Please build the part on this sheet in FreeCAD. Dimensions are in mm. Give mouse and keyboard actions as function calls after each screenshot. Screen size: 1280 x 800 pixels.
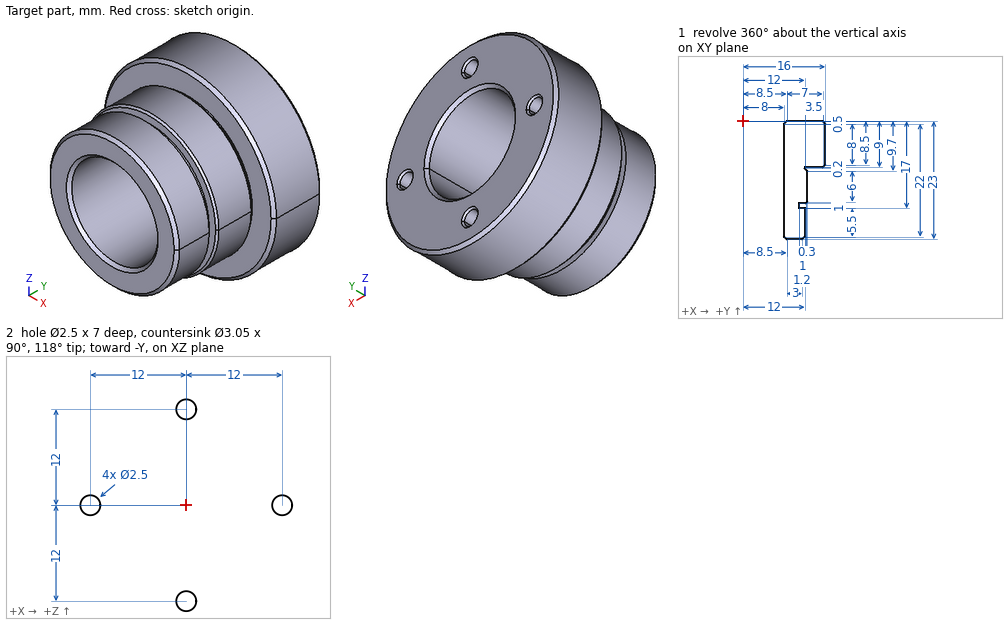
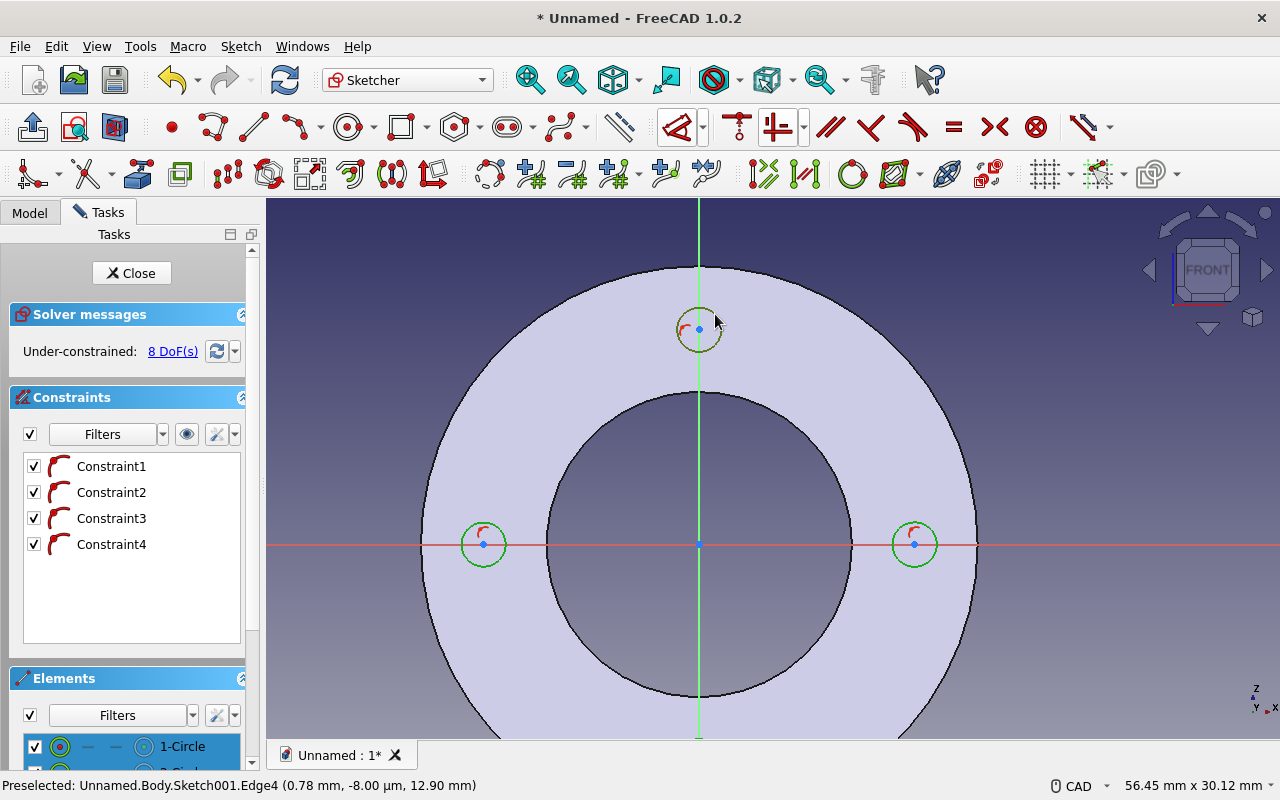
key(e)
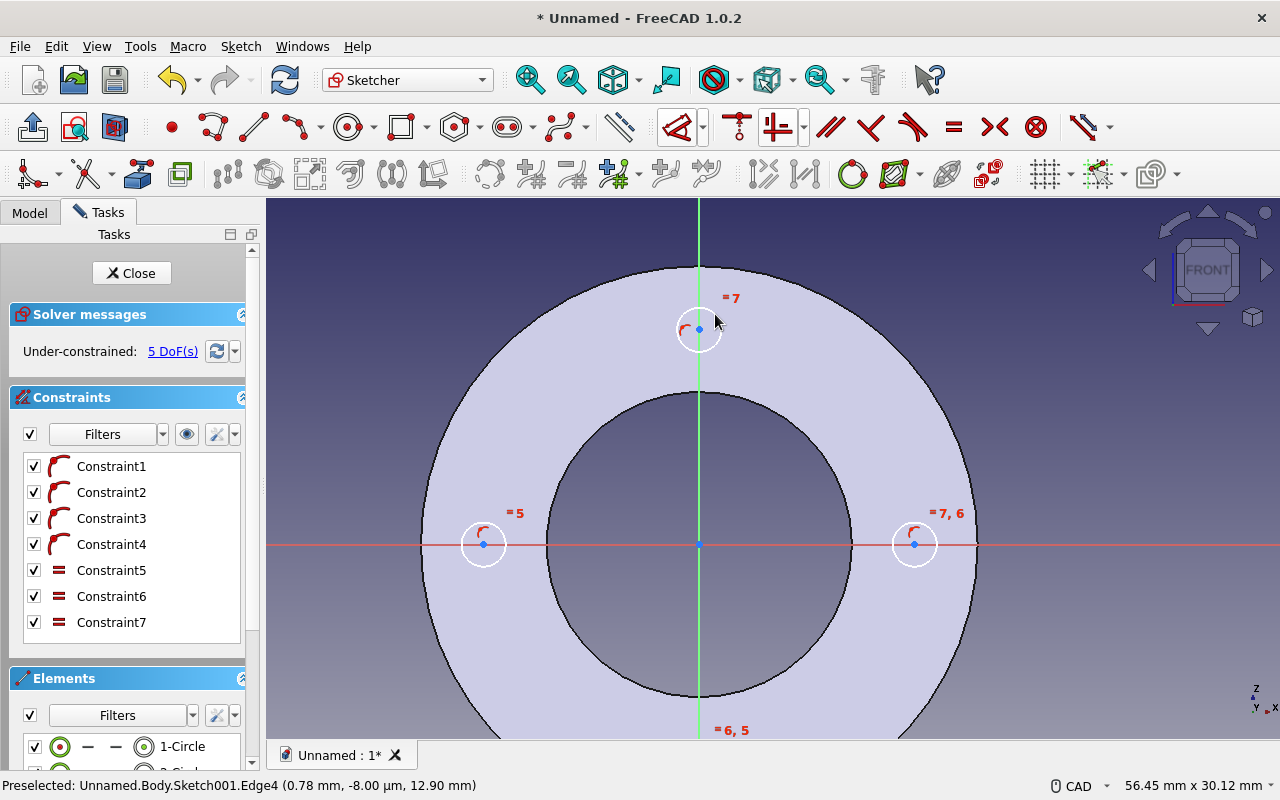
click(676, 128)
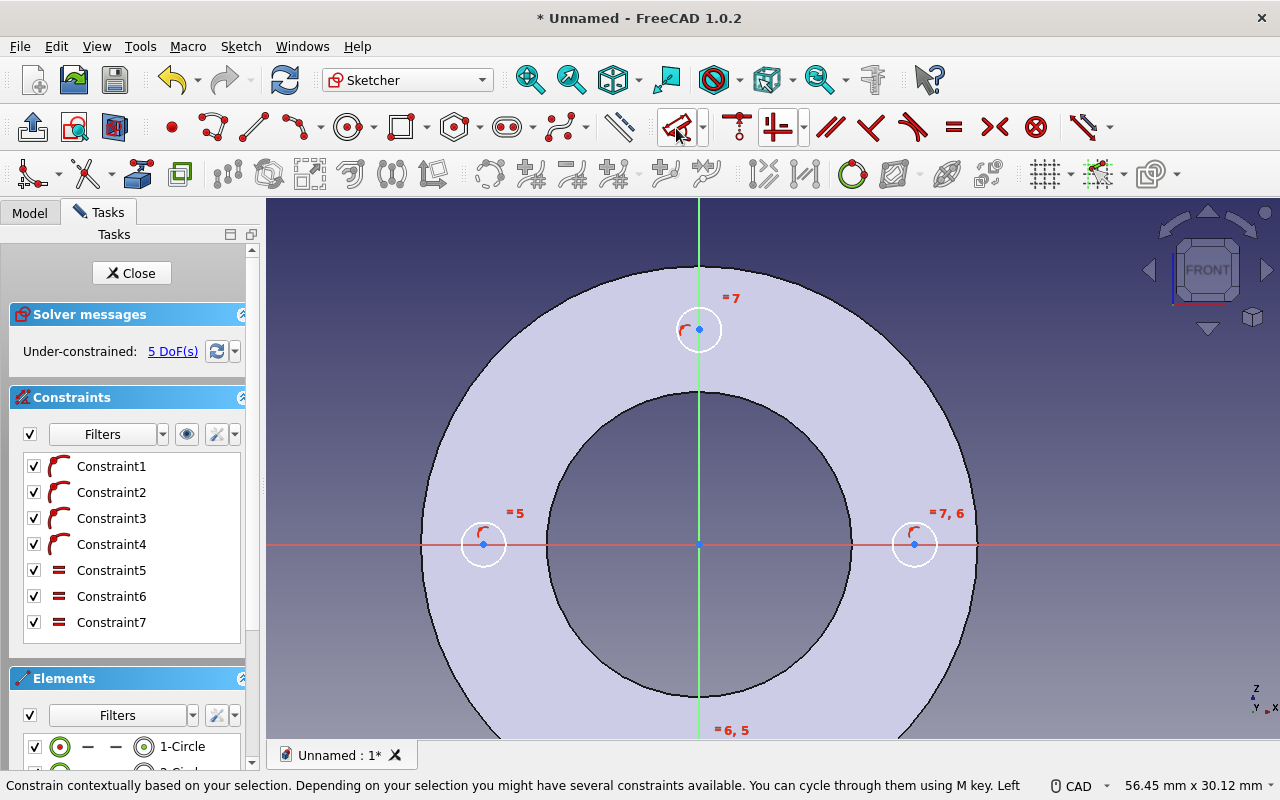
click(499, 529)
click(522, 506)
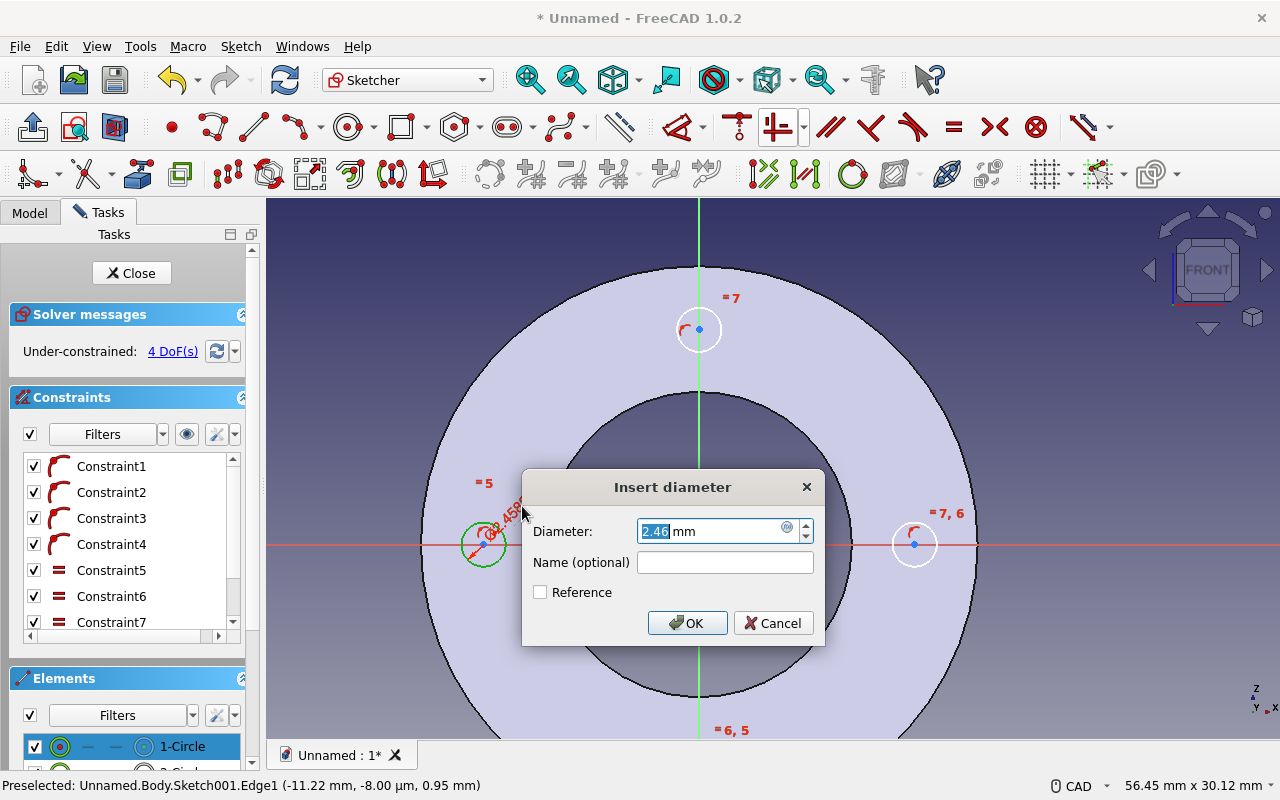
text(2.5)
key(Return)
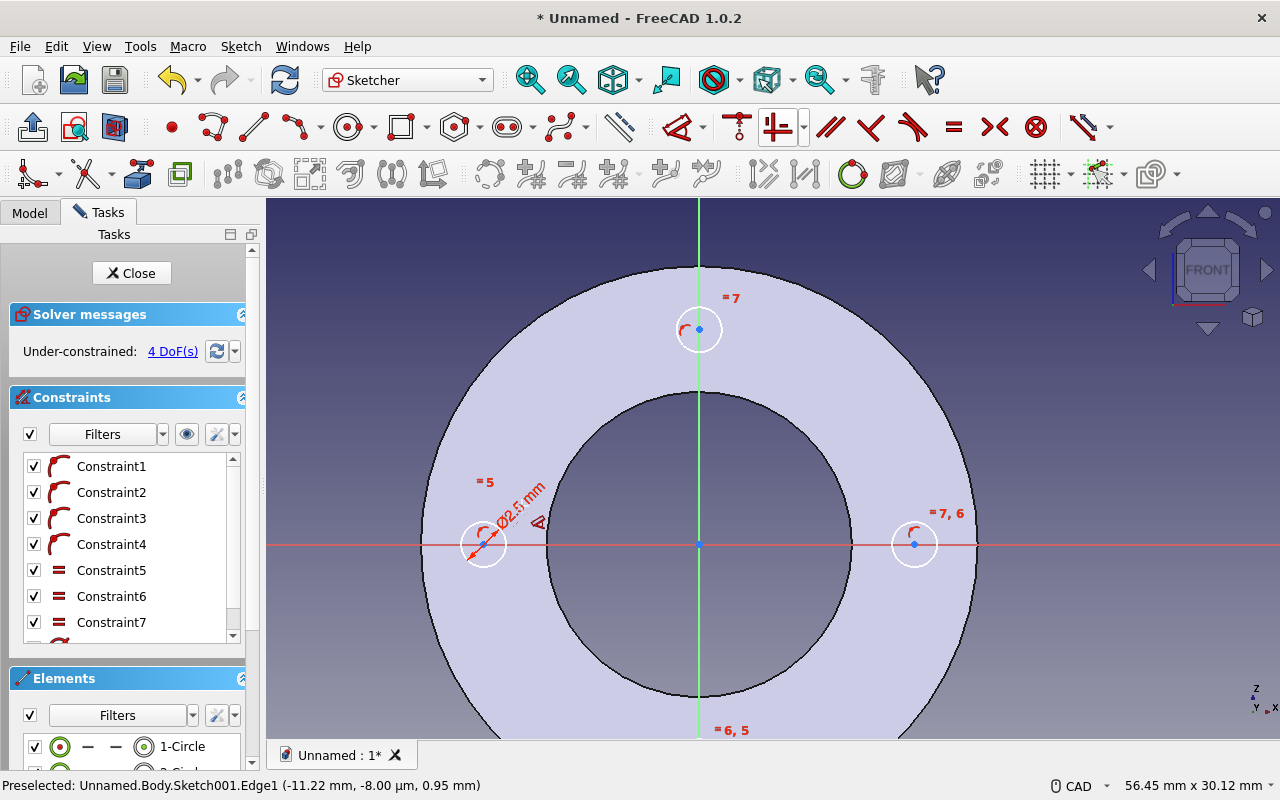
click(484, 545)
click(591, 579)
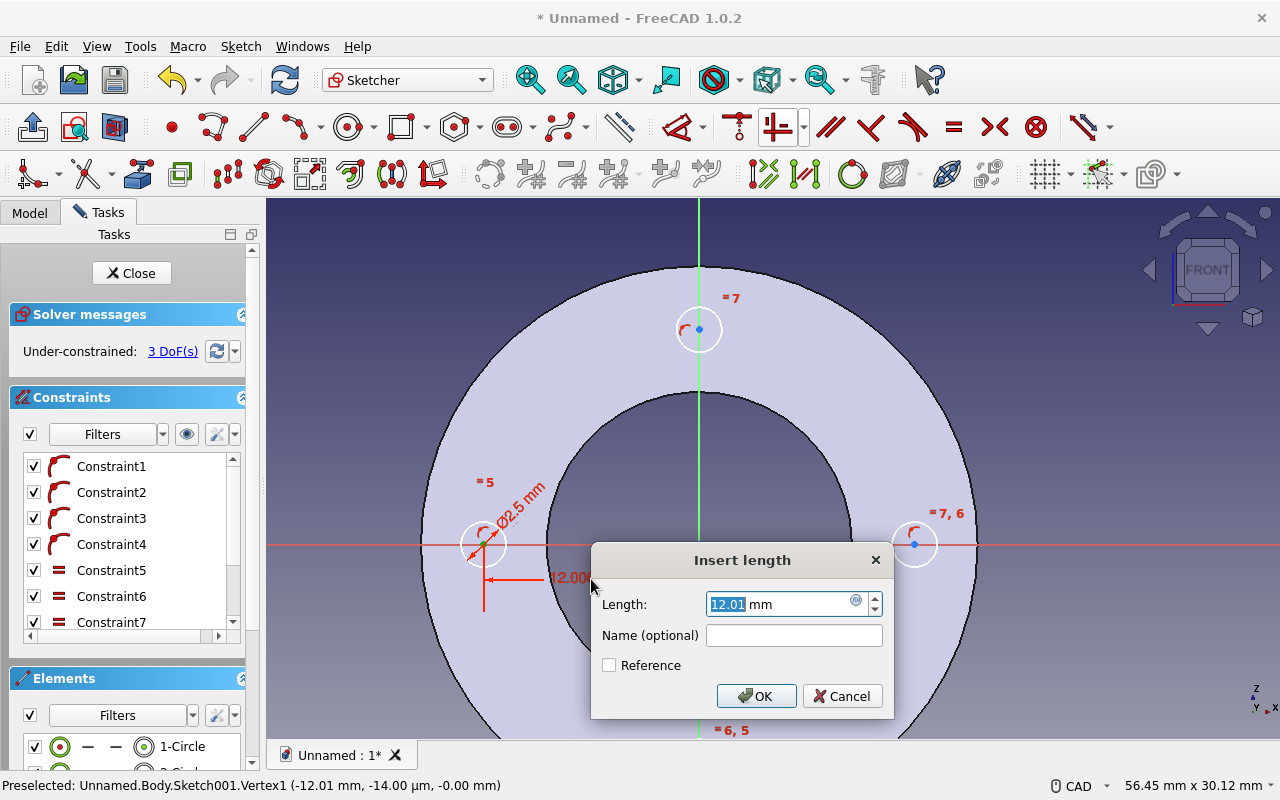
text(12)
key(Return)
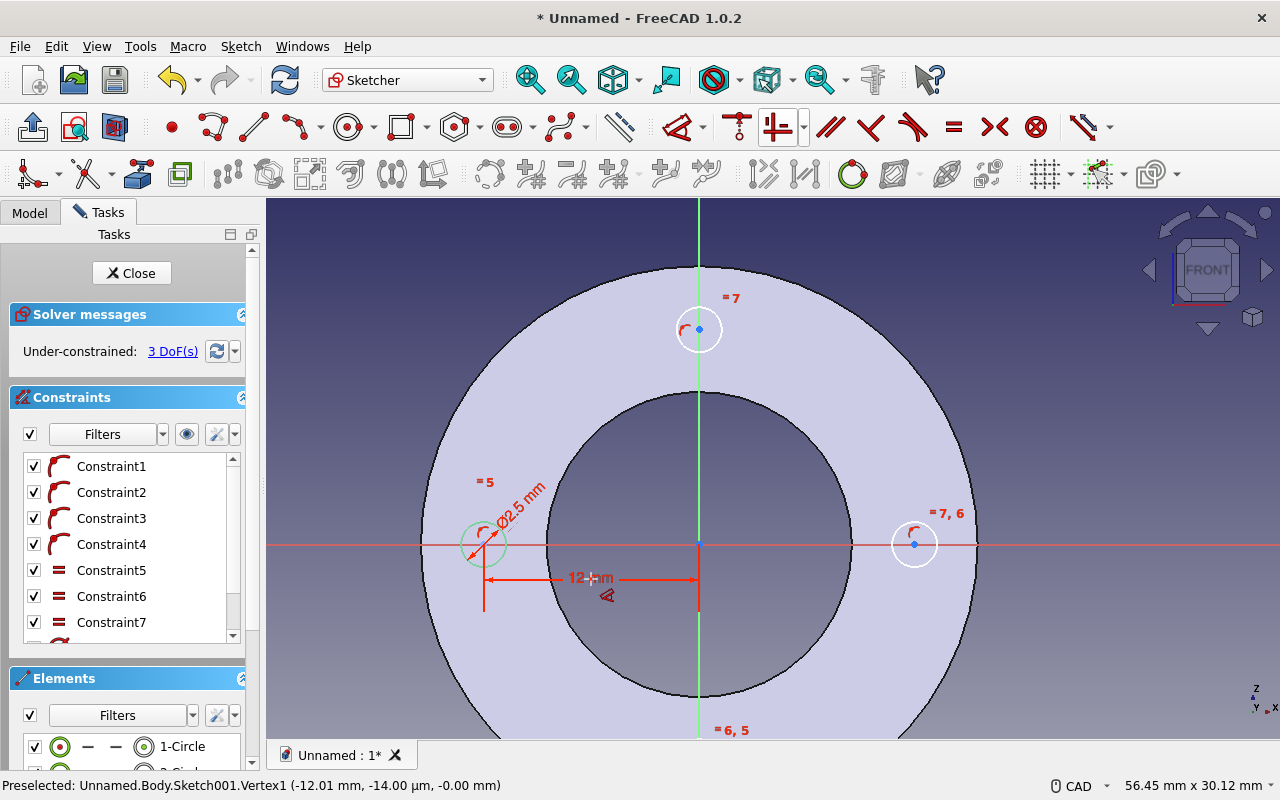
scroll(715, 314, down, 2)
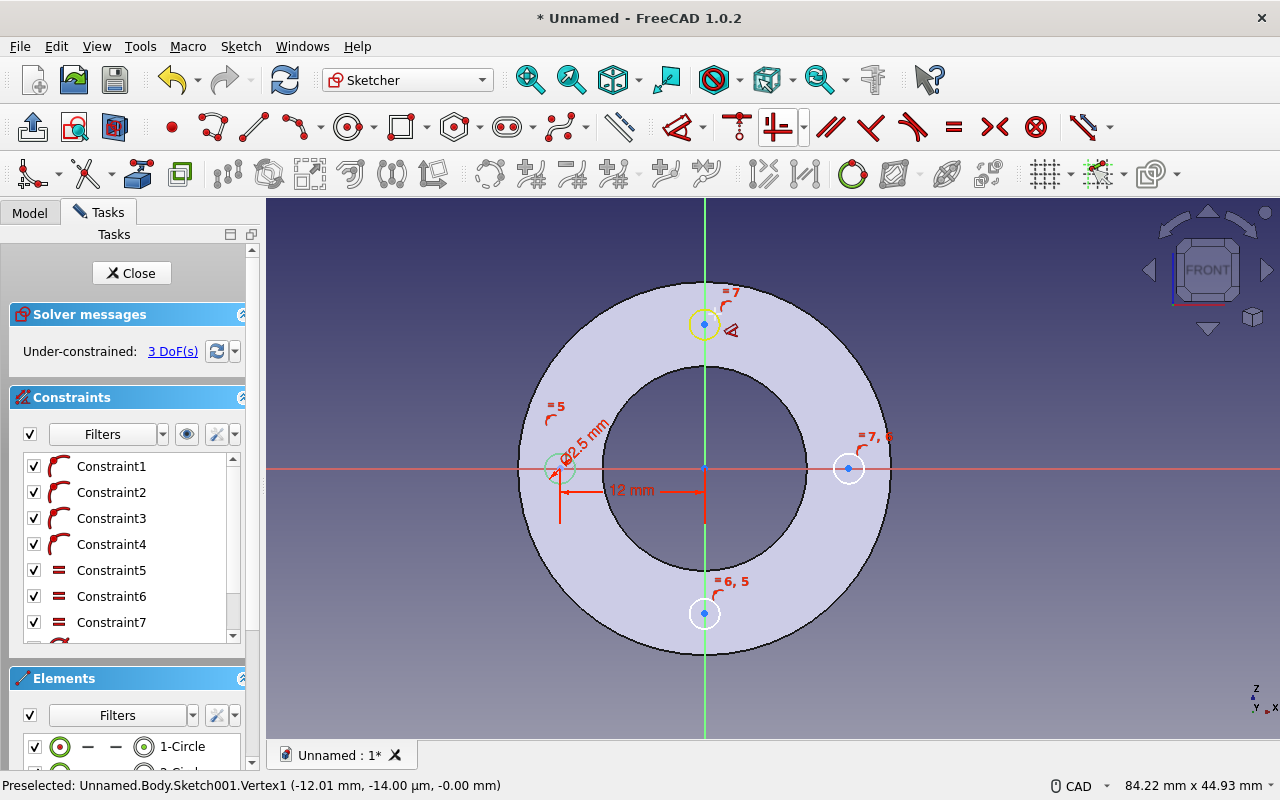
click(705, 614)
click(739, 541)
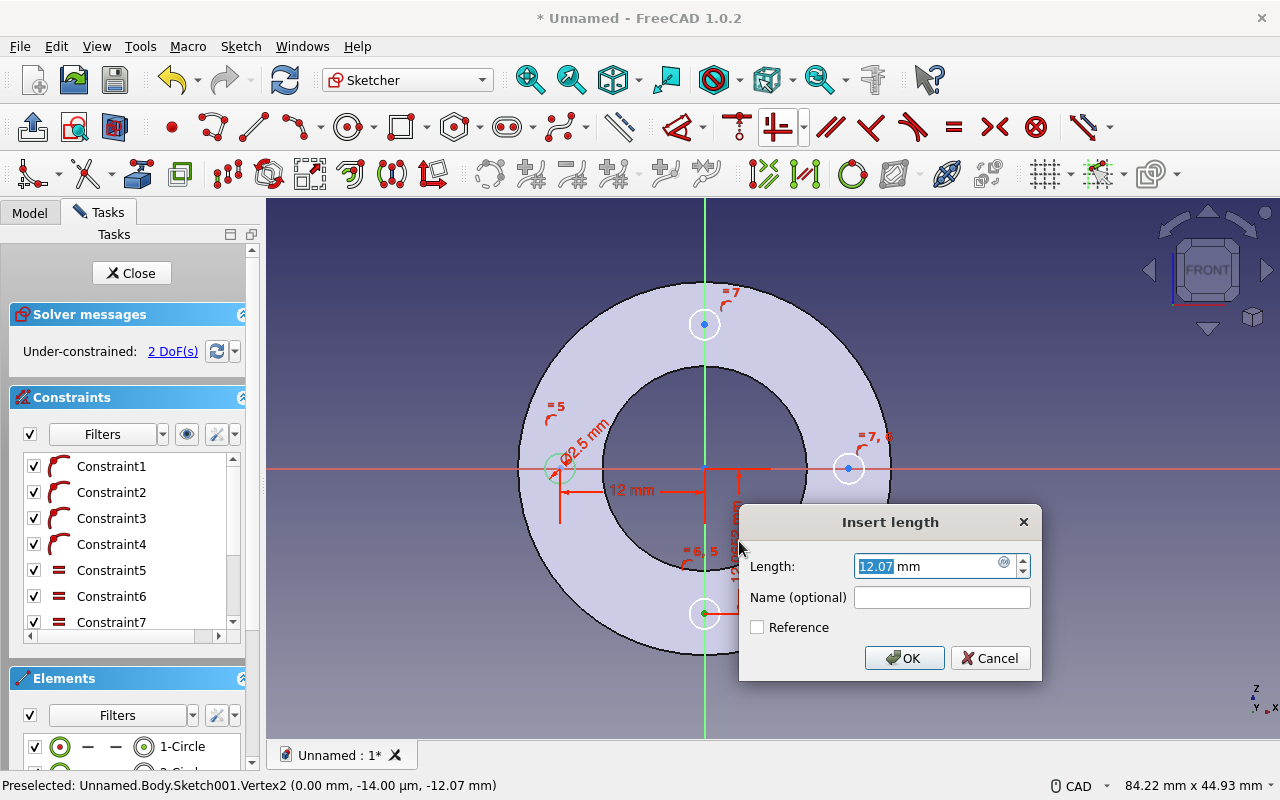
text(12)
key(Return)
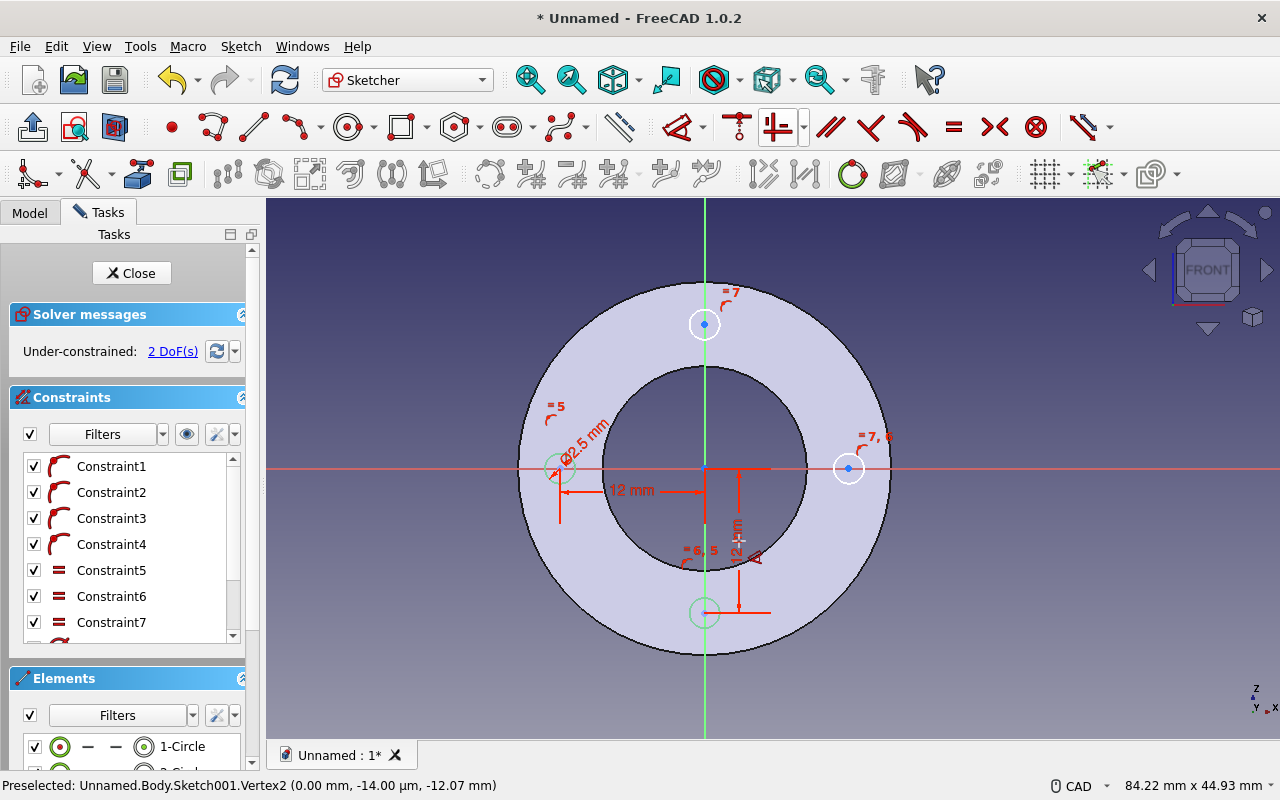
click(849, 469)
click(777, 503)